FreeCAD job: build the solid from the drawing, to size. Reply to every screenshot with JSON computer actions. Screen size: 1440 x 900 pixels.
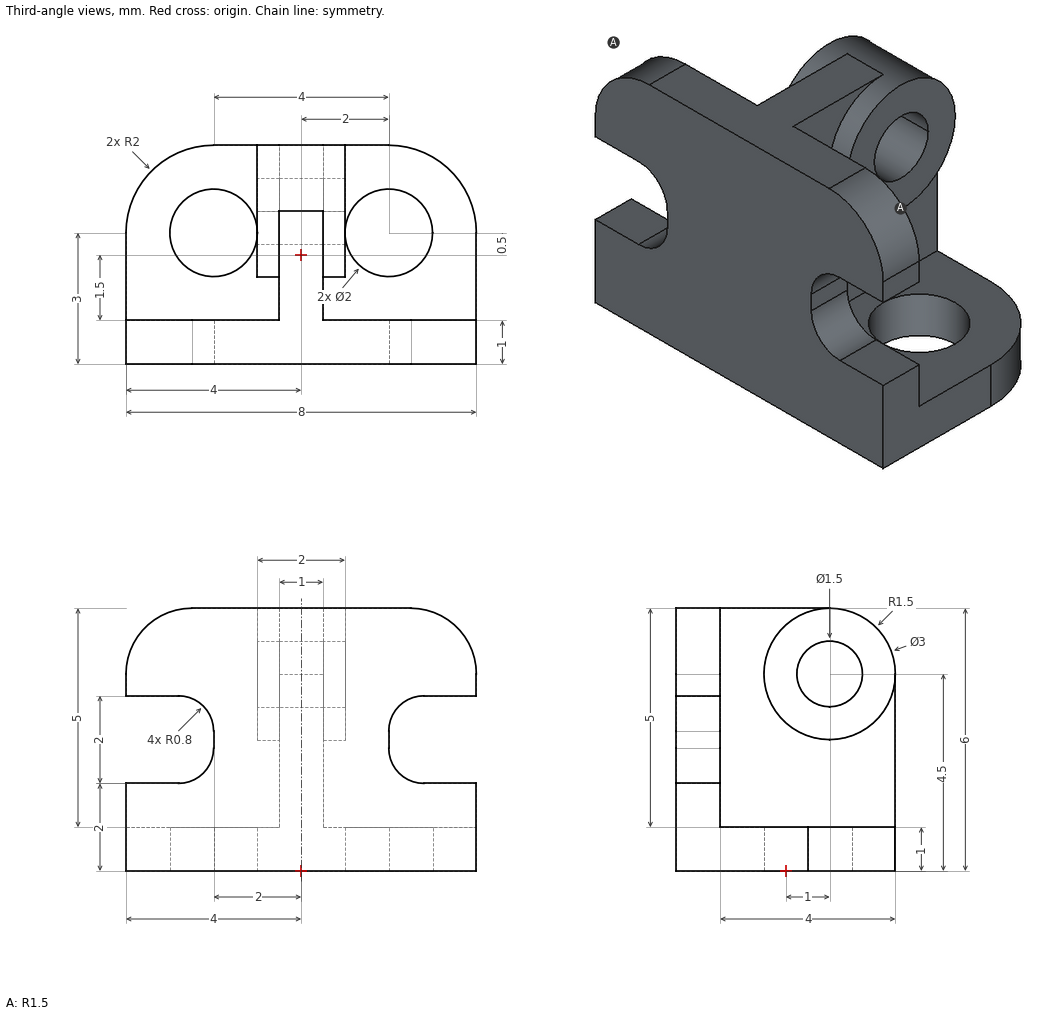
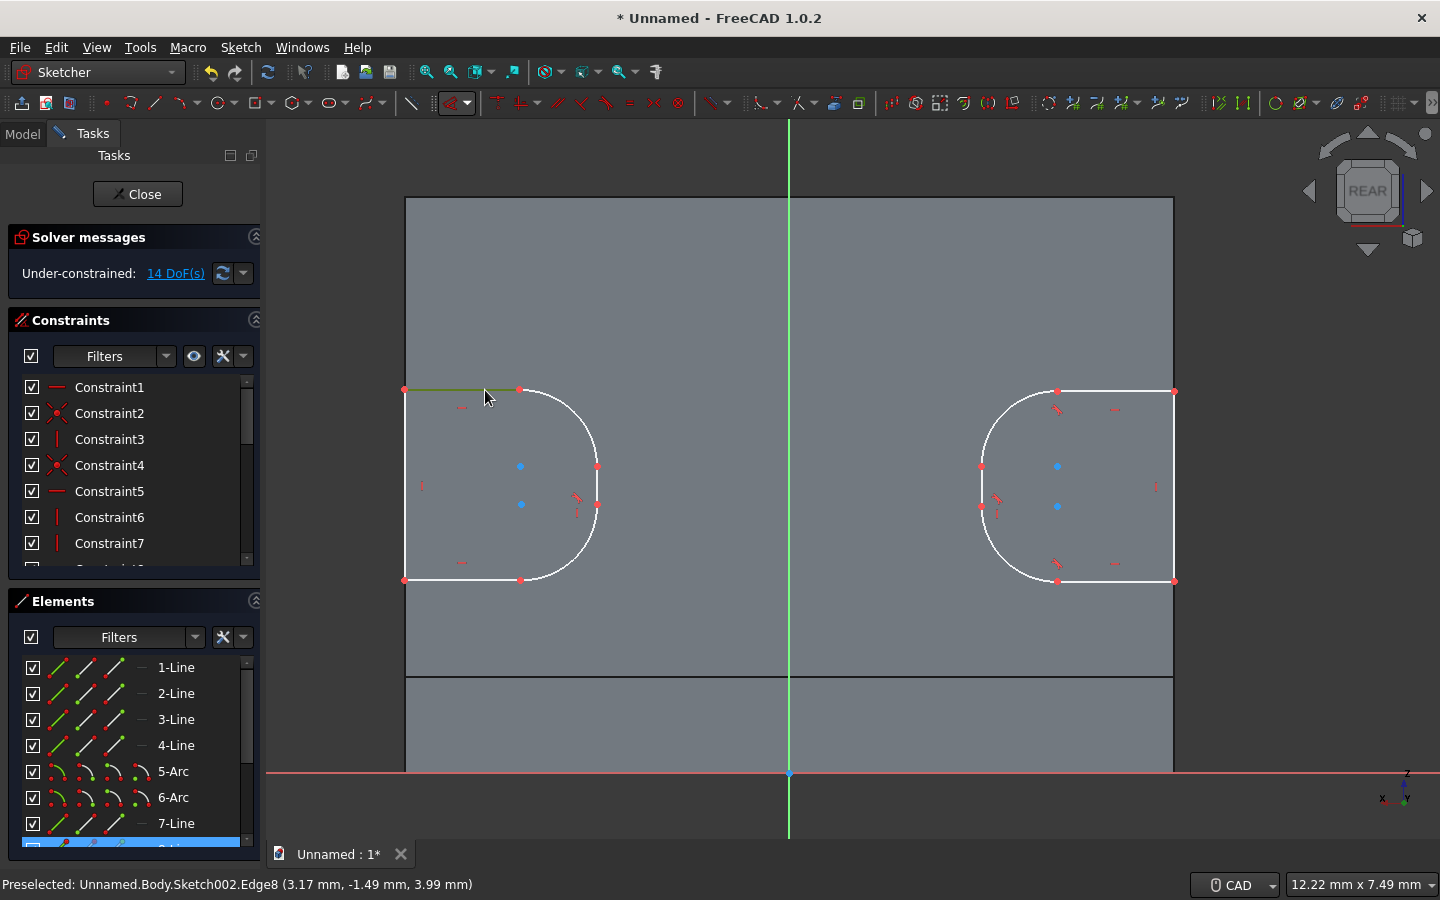
{"action": "left_click", "coordinate": [589, 432]}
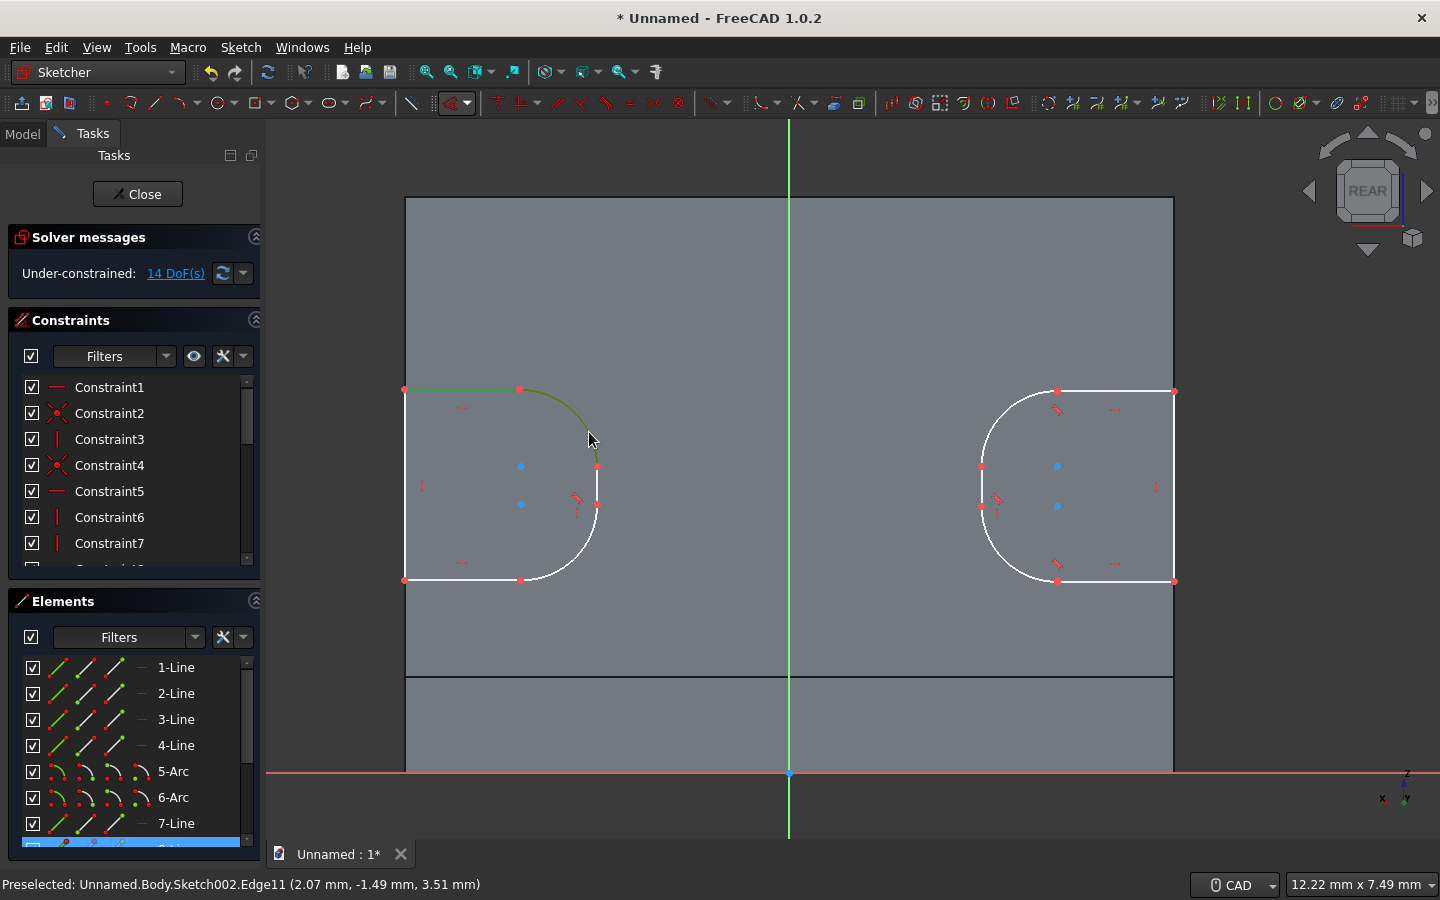
{"action": "left_click", "coordinate": [606, 104]}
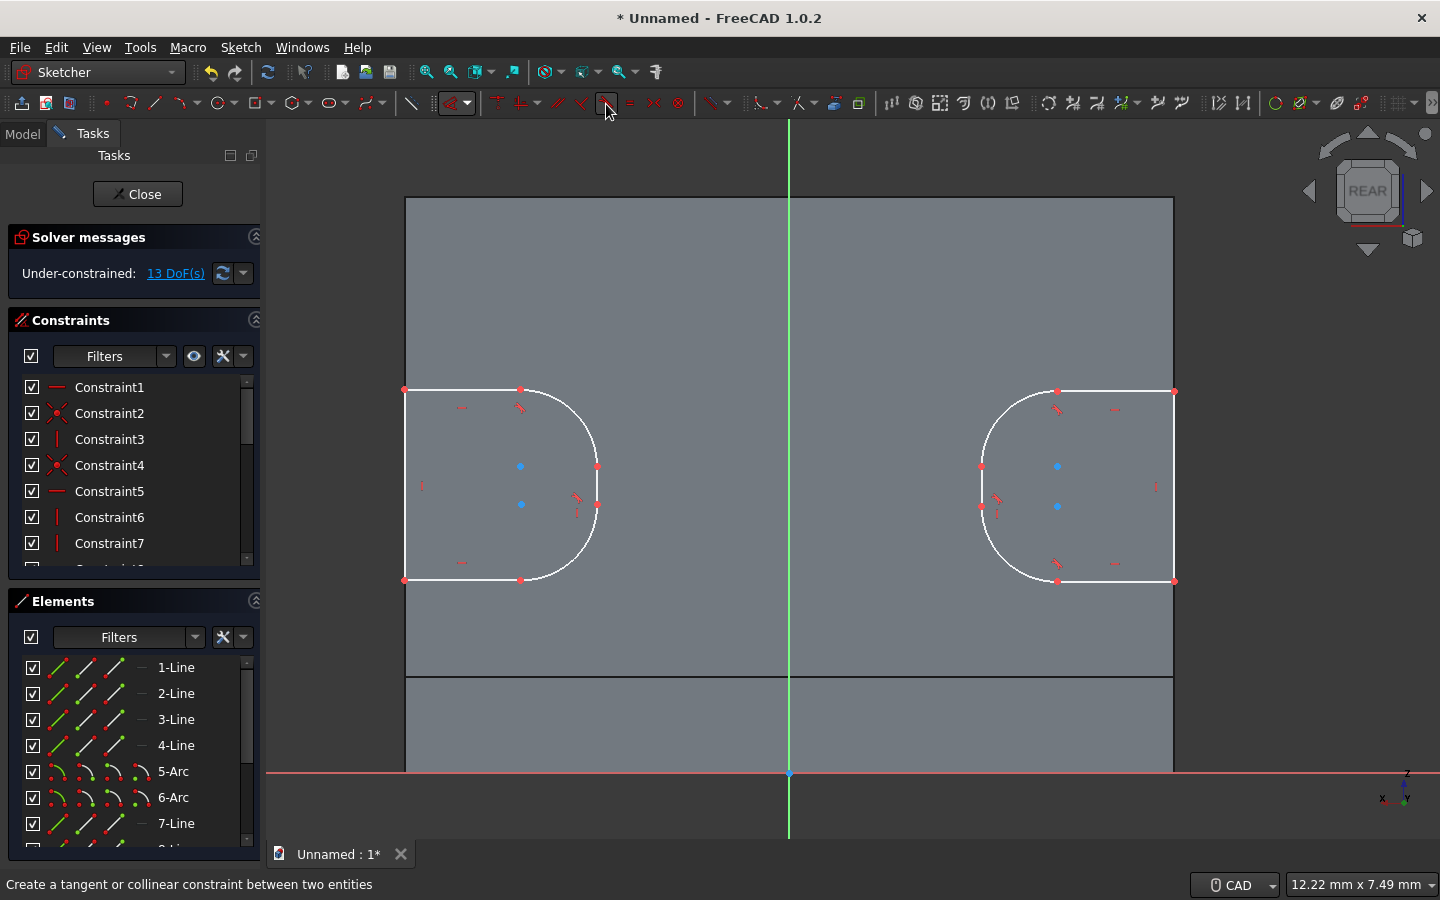
{"action": "left_click", "coordinate": [440, 580]}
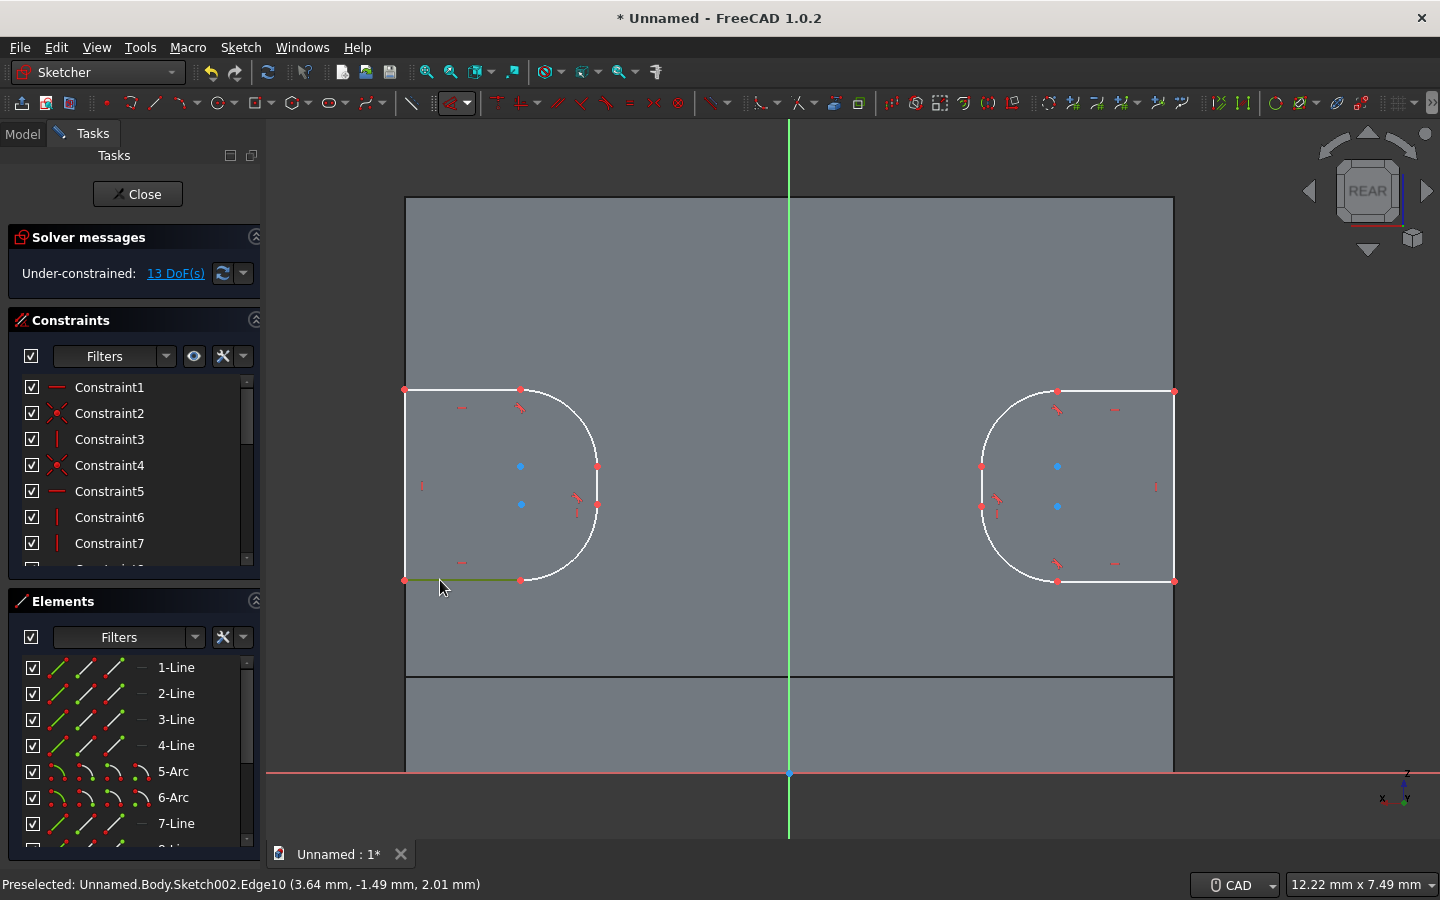
{"action": "left_click", "coordinate": [555, 573]}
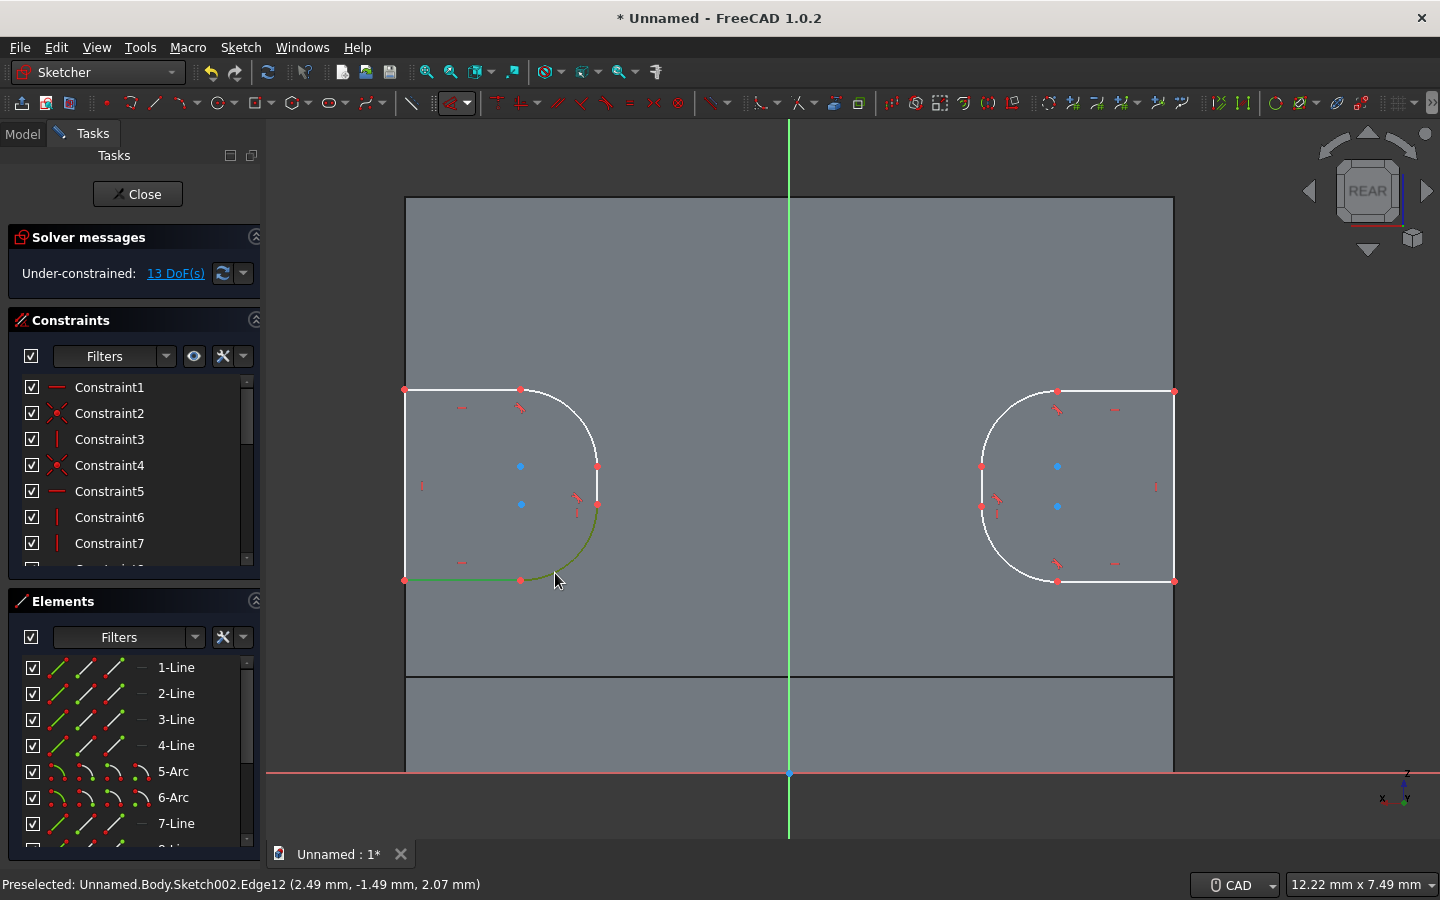
{"action": "left_click", "coordinate": [606, 104]}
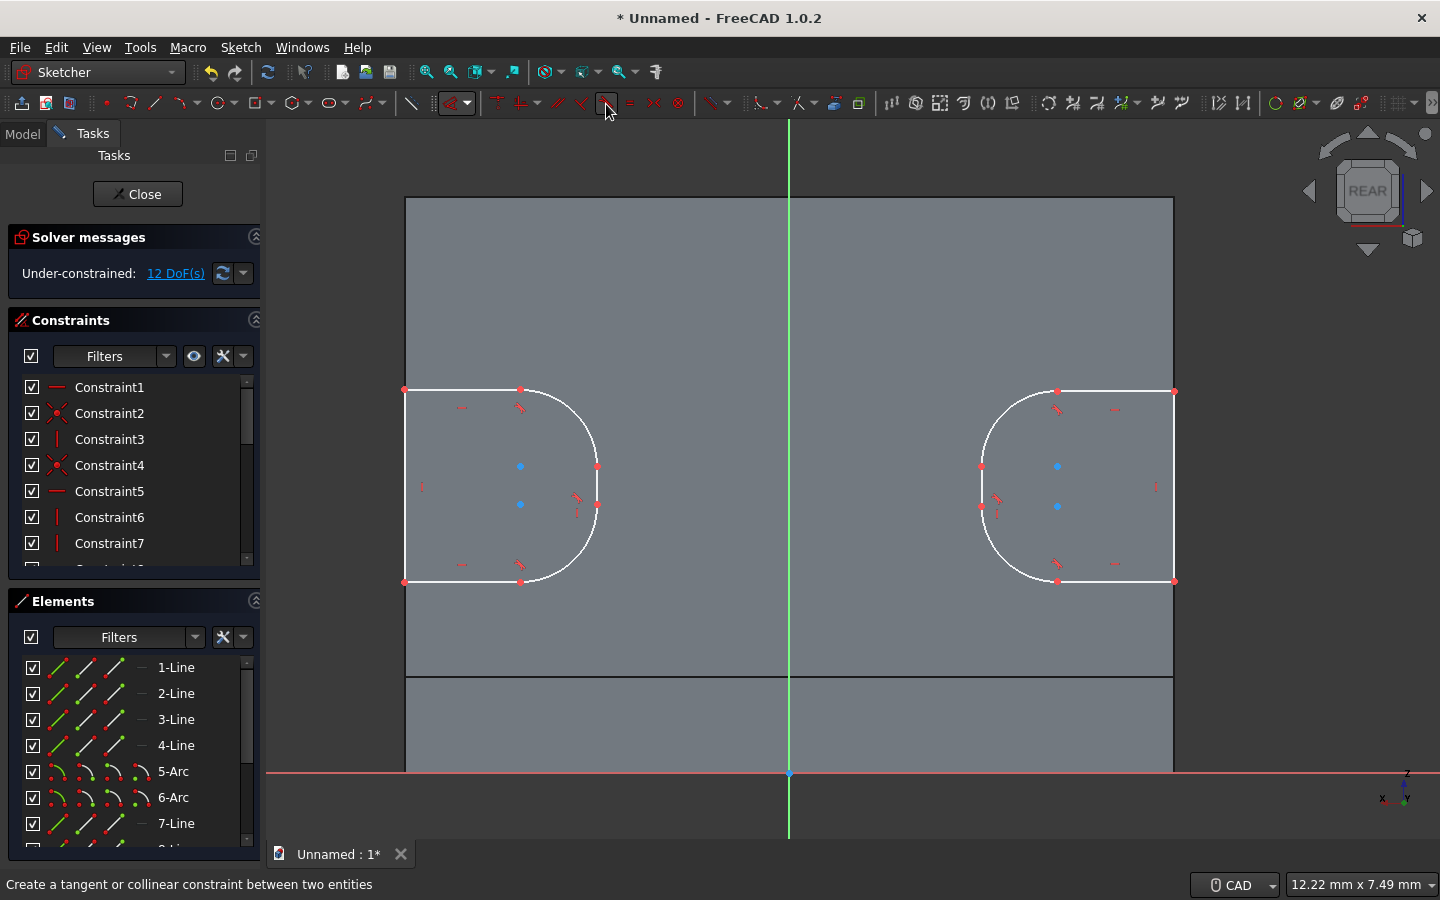
{"action": "left_click", "coordinate": [1023, 399]}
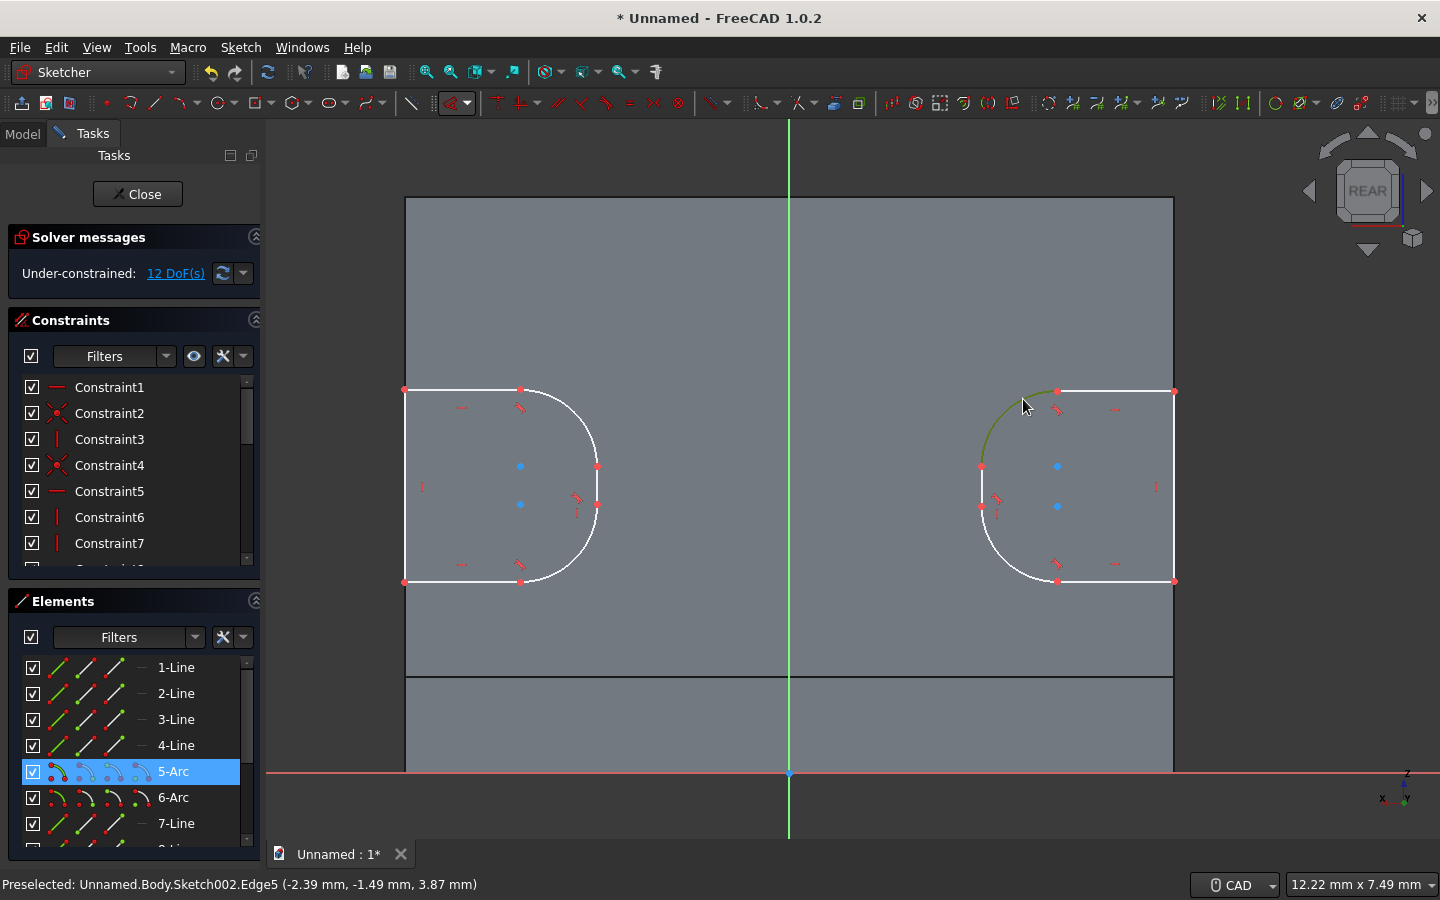
{"action": "left_click", "coordinate": [990, 540]}